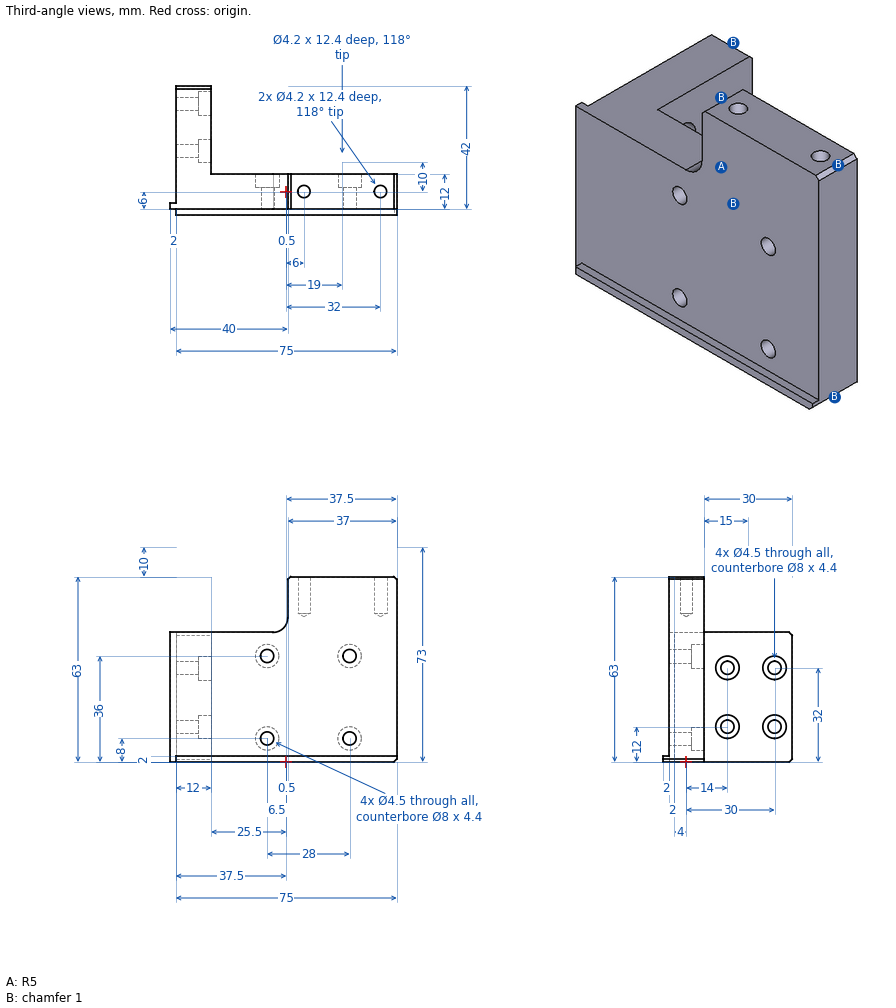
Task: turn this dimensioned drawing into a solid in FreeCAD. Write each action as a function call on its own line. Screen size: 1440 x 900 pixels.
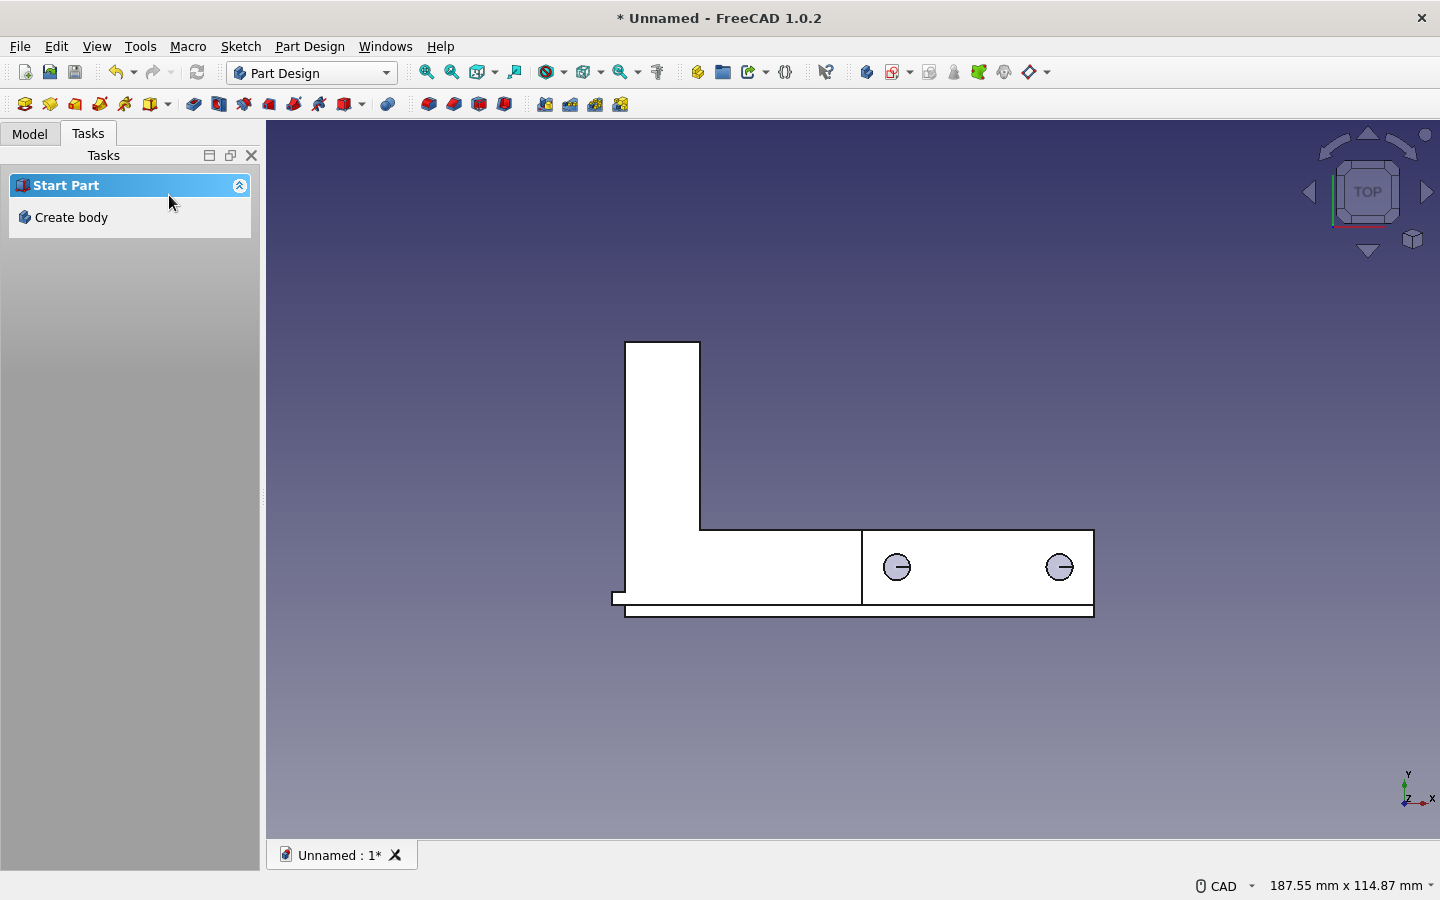
click(427, 72)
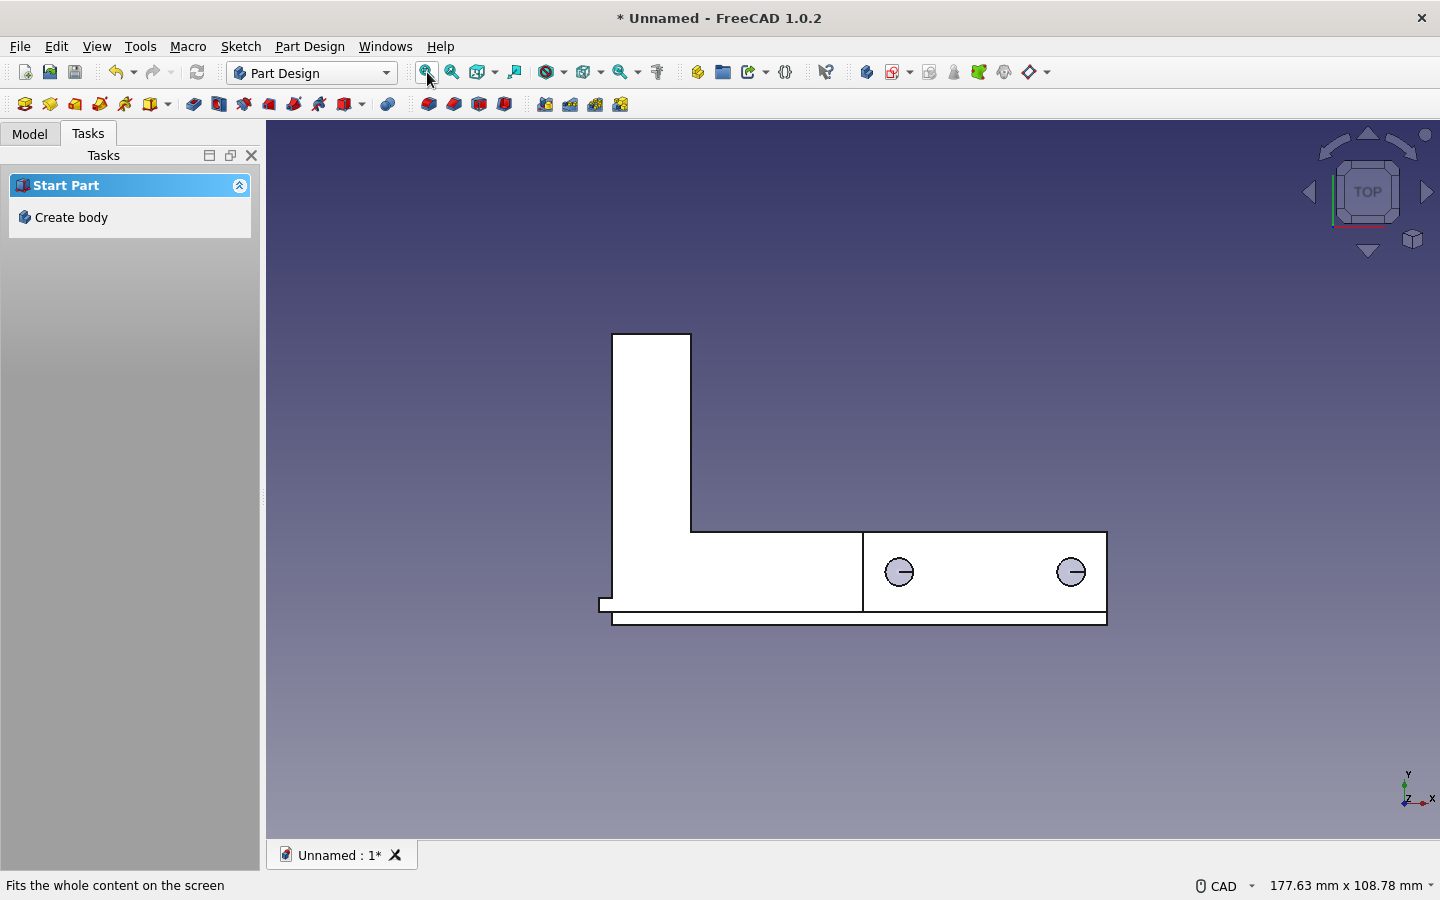
key(0)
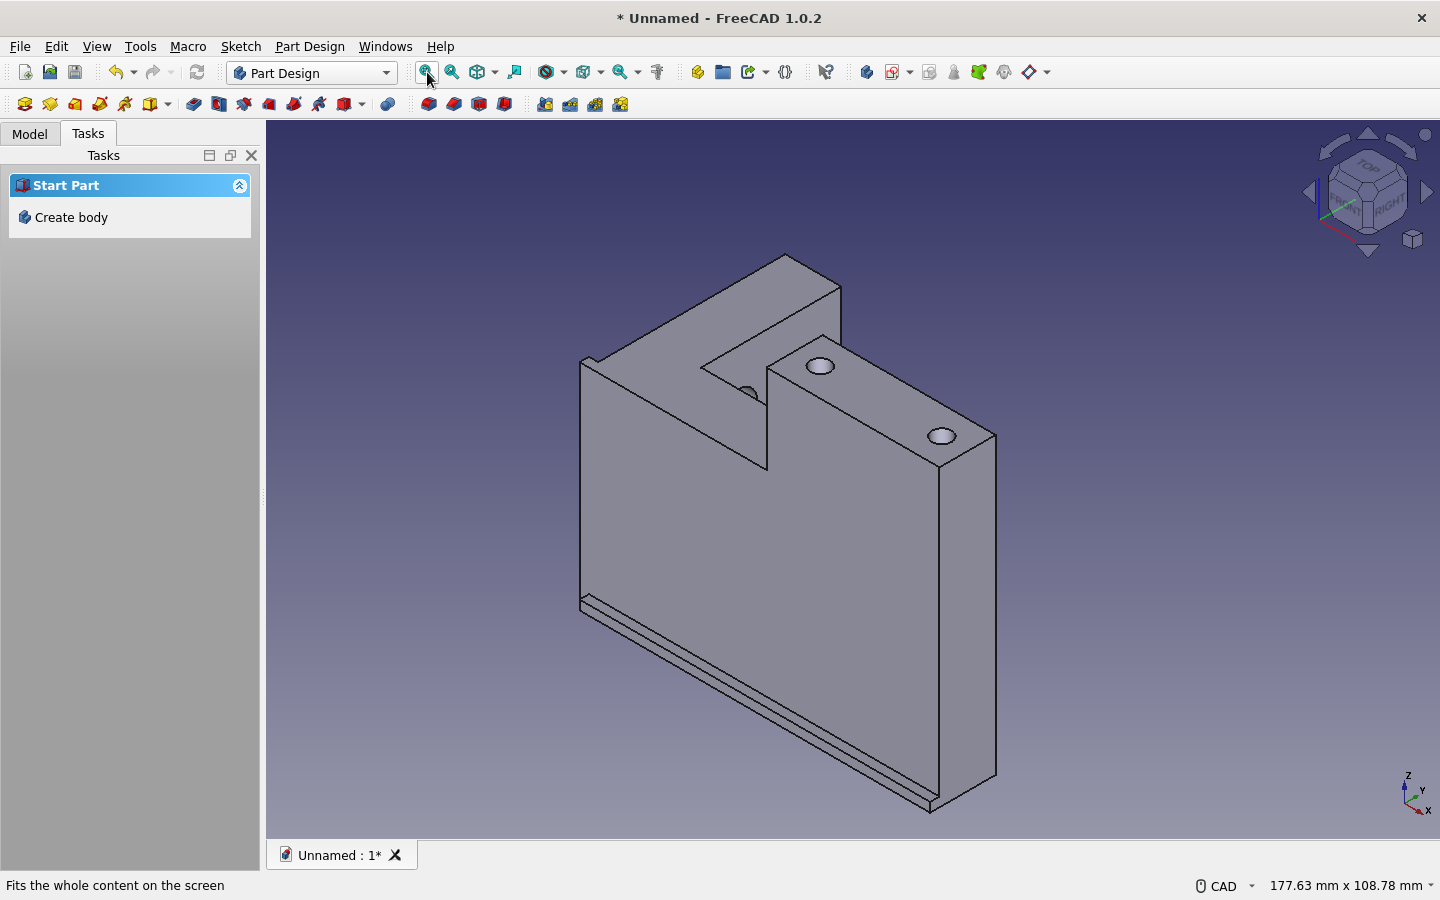
key(1)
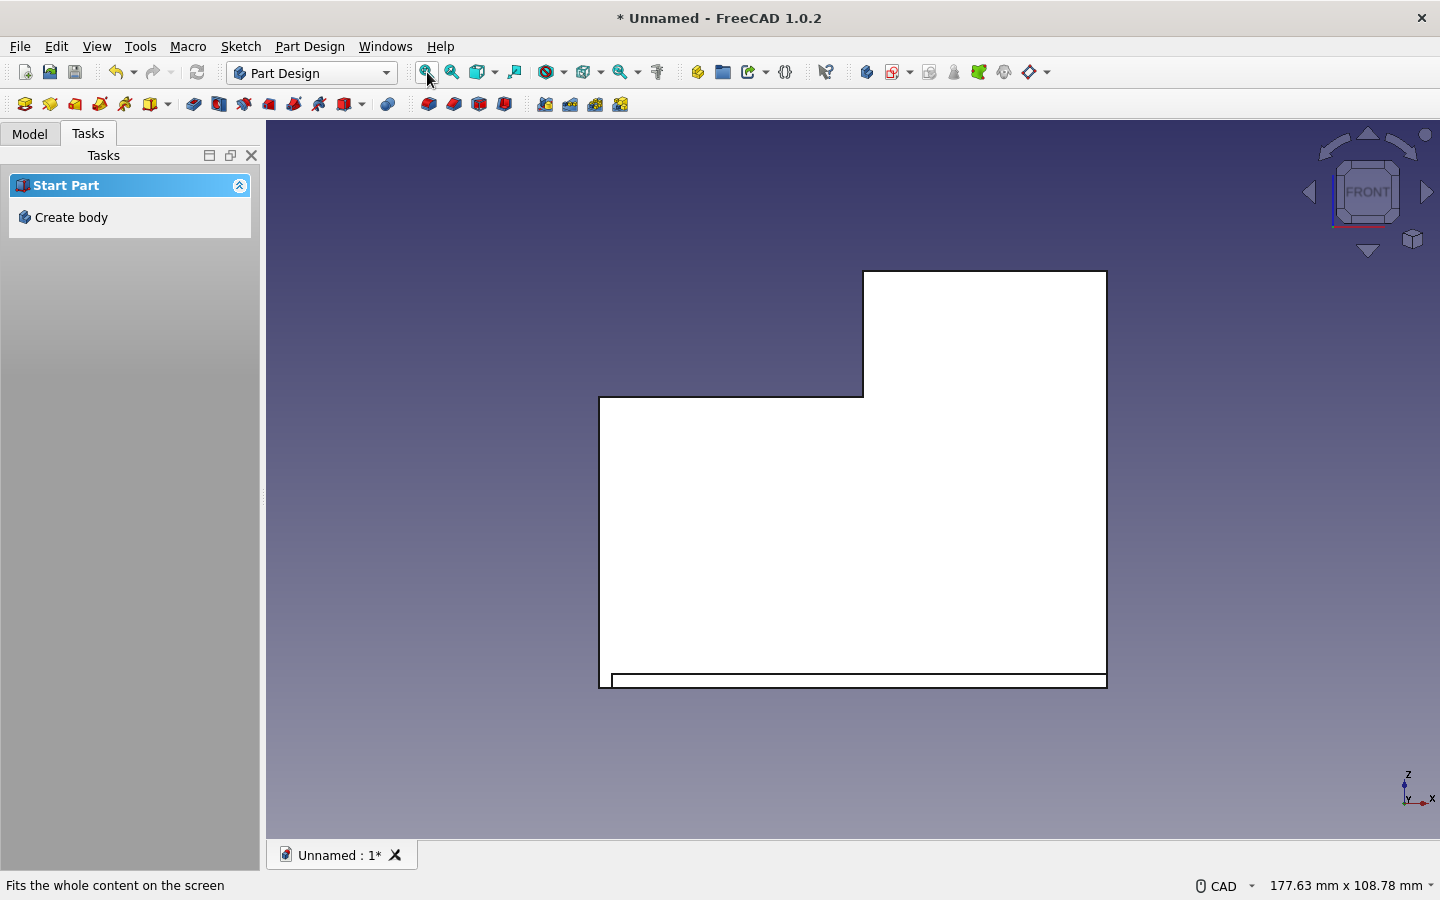
key(3)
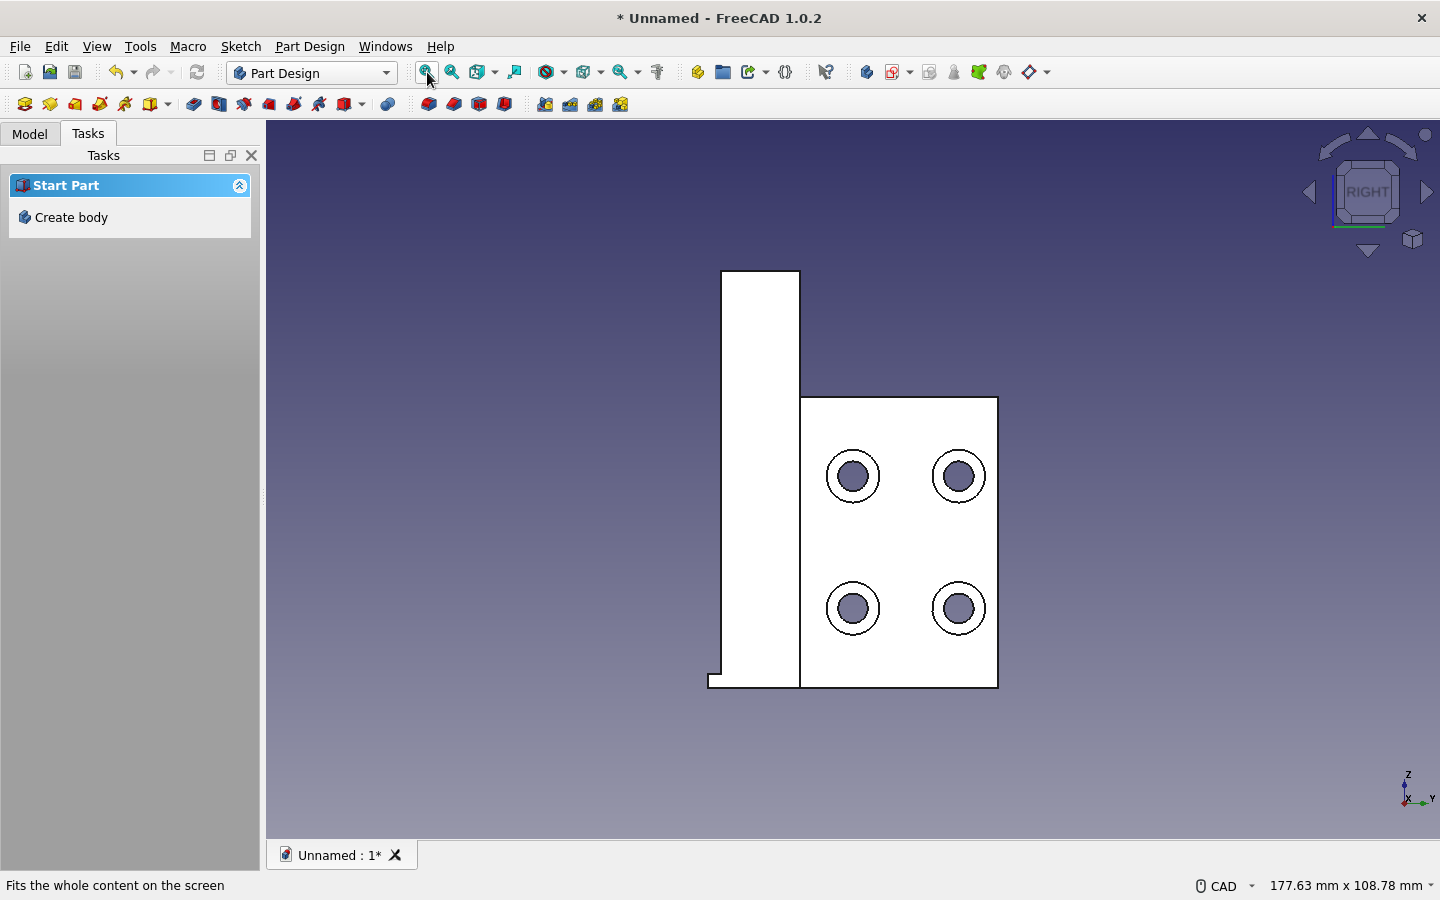
key(5)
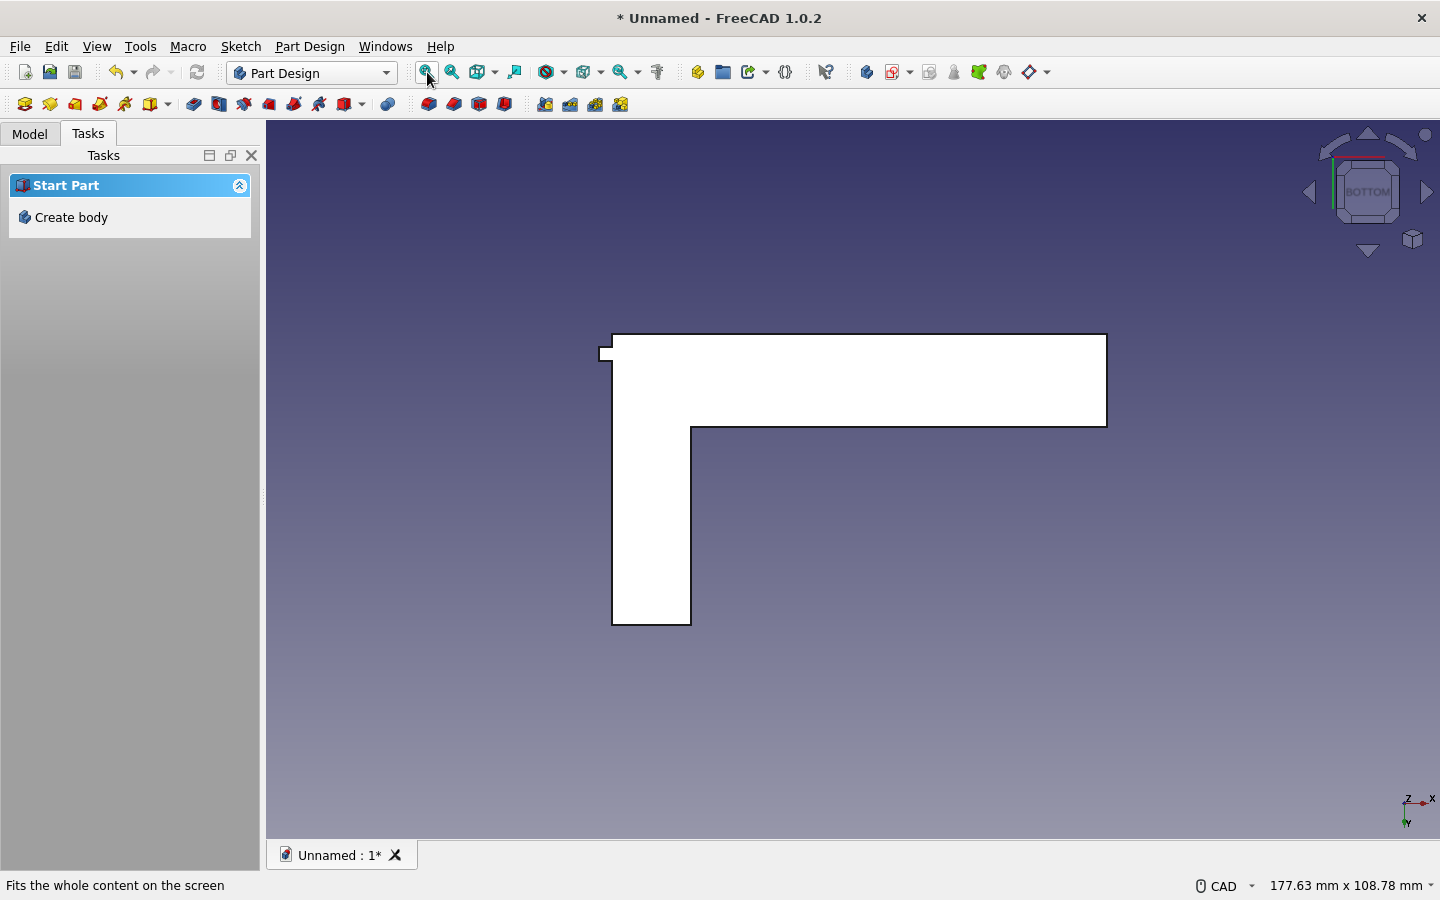
click(427, 72)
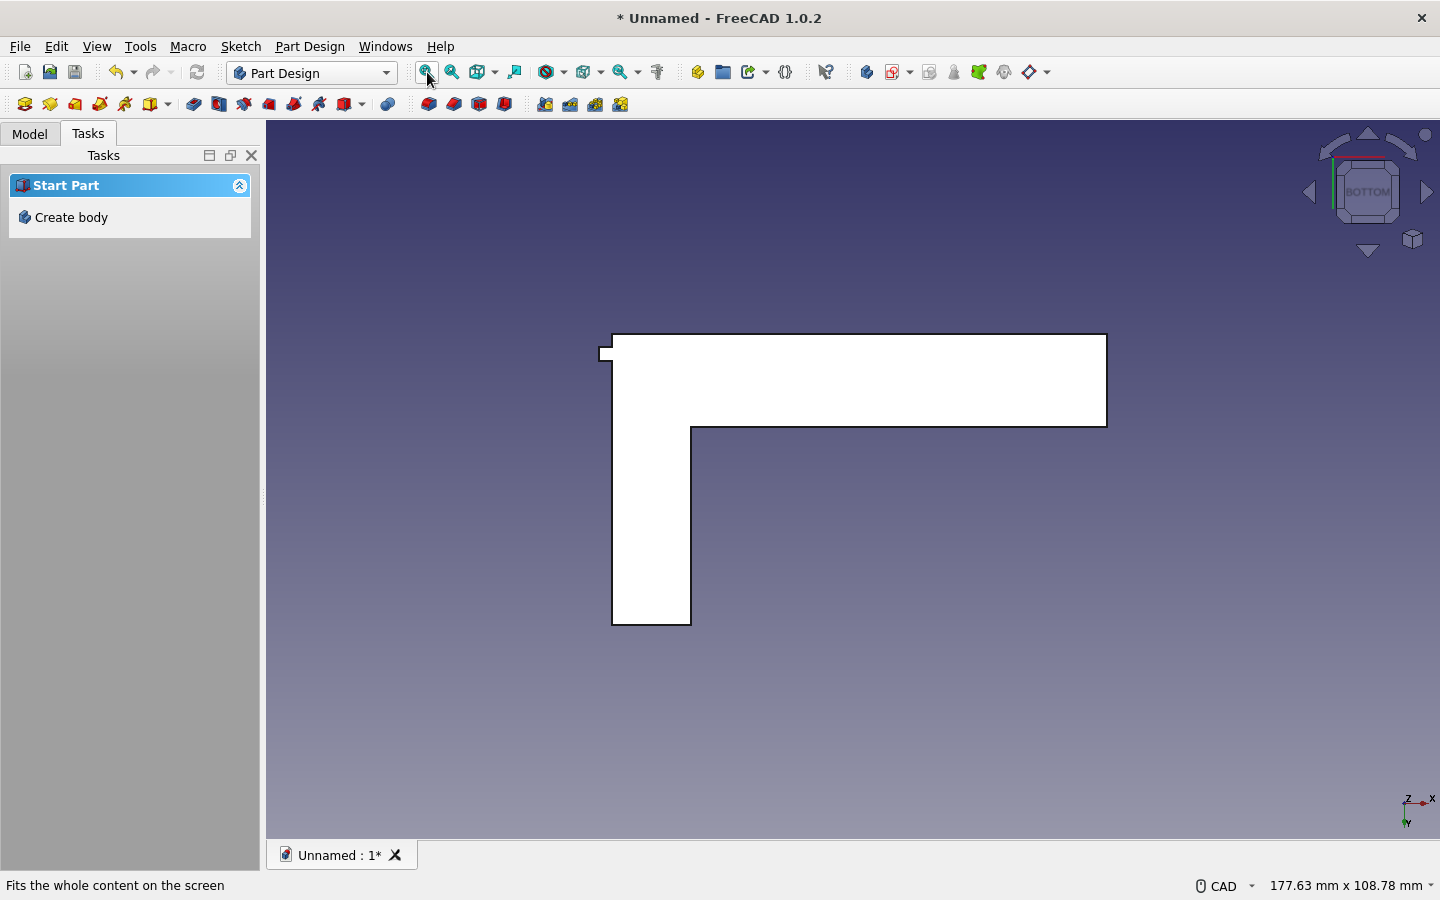
key(4)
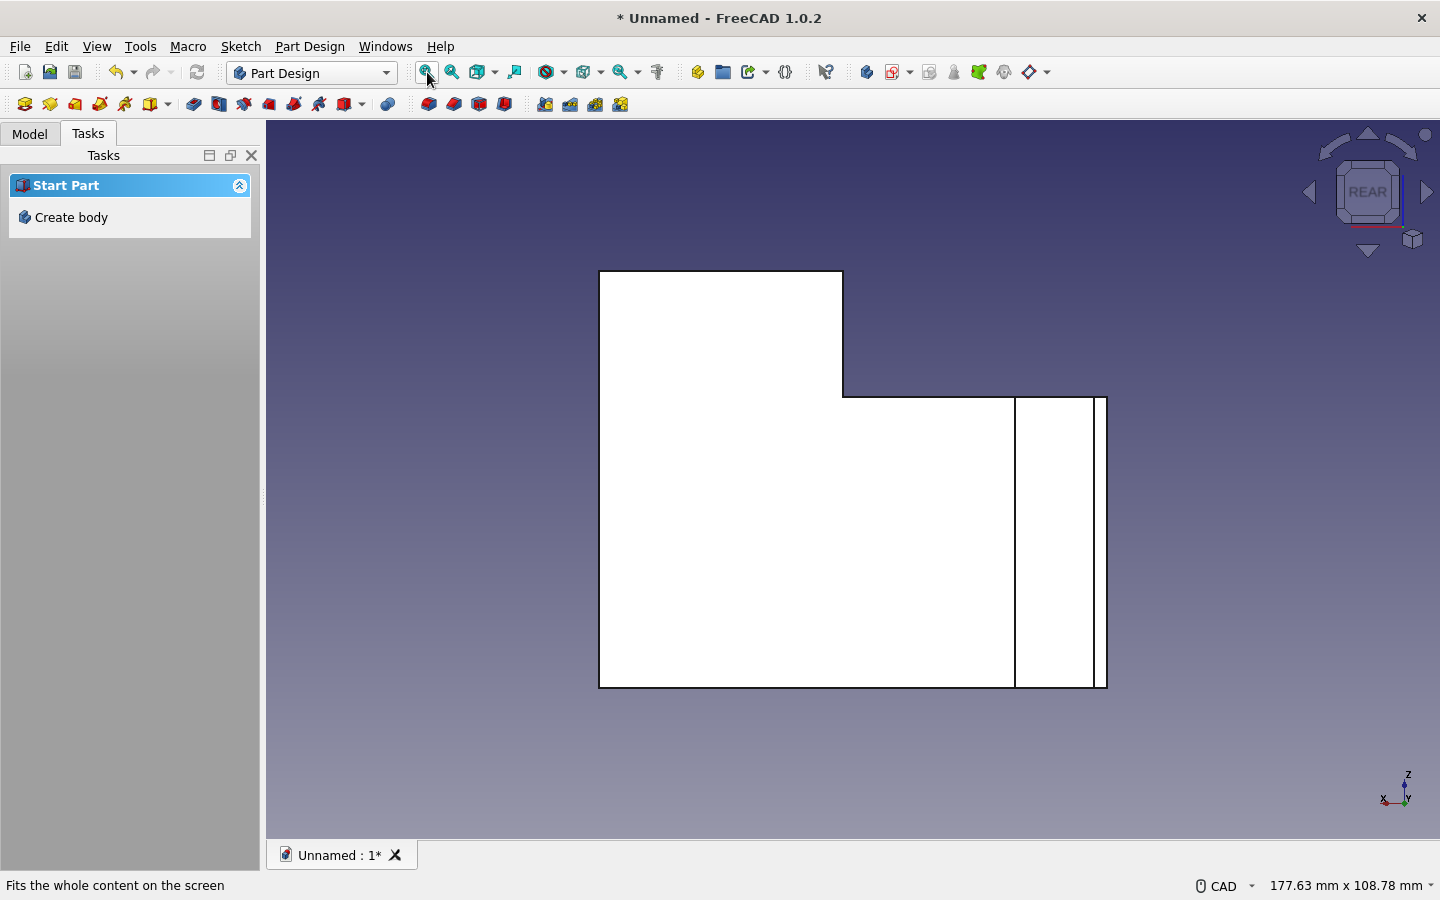
key(6)